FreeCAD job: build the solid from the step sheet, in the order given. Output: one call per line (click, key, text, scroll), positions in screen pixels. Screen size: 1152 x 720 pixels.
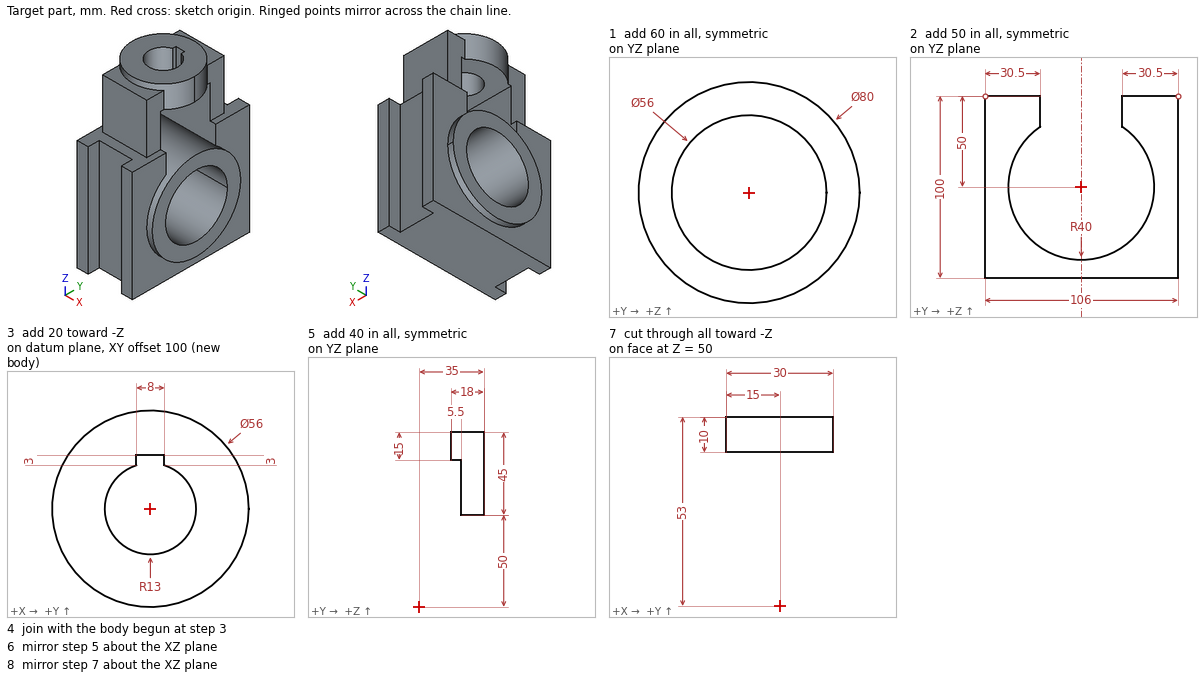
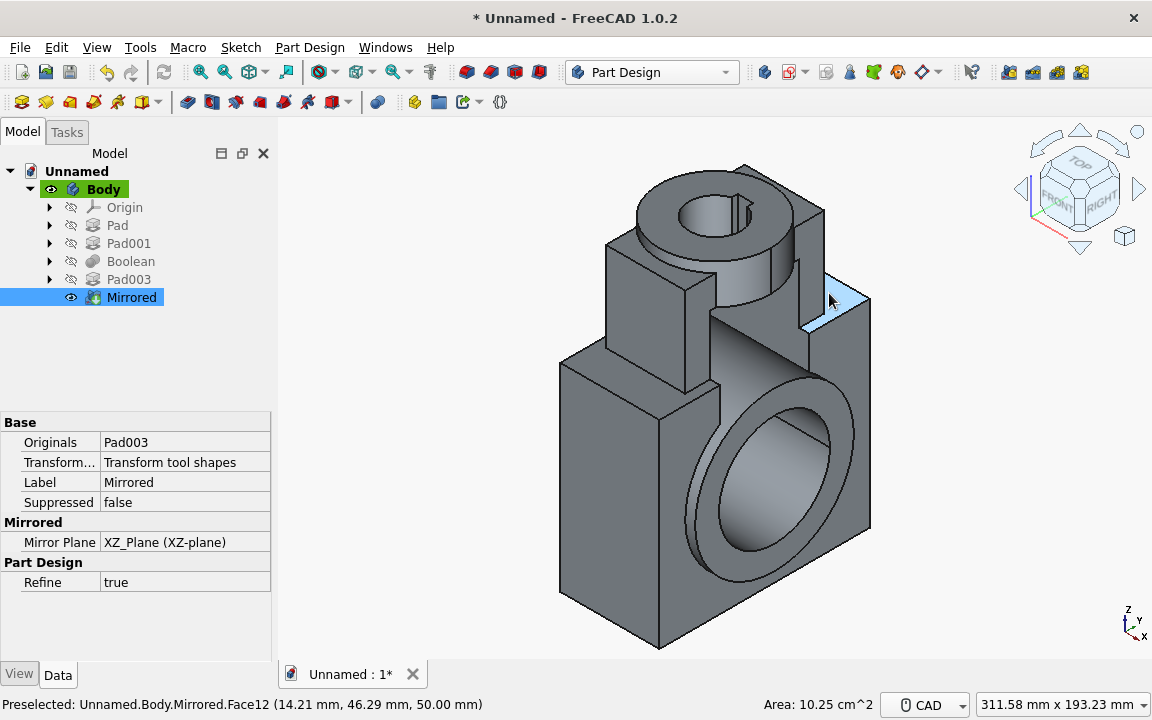
click(790, 72)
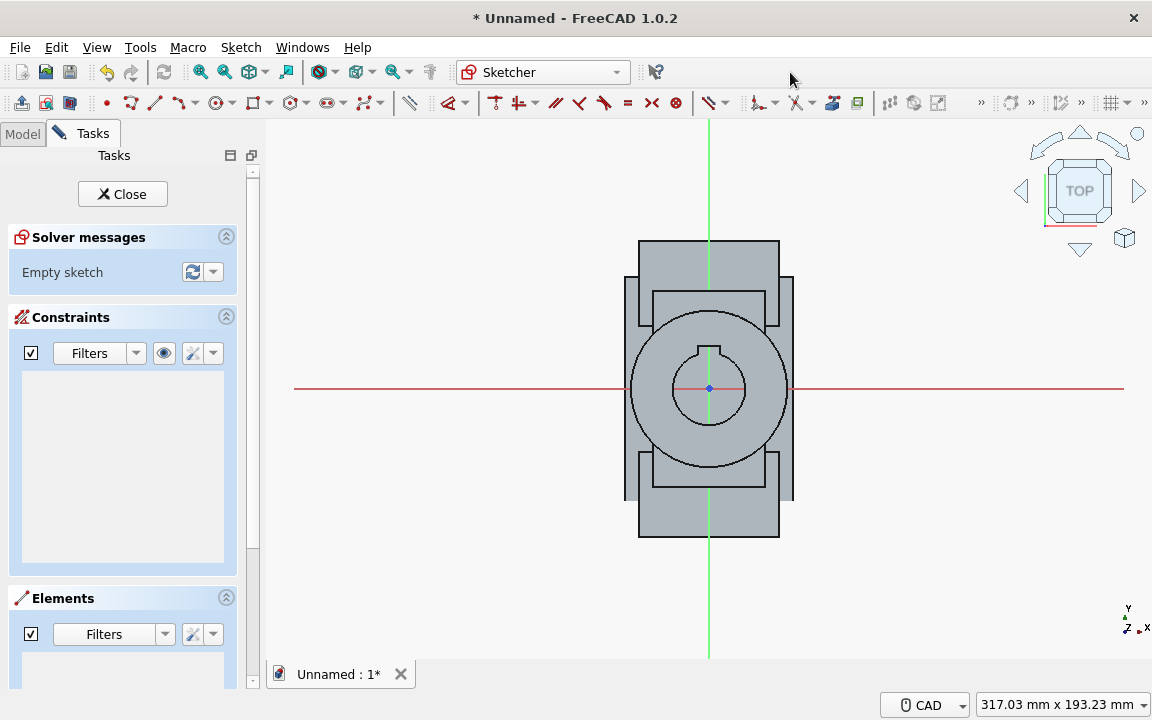
click(70, 104)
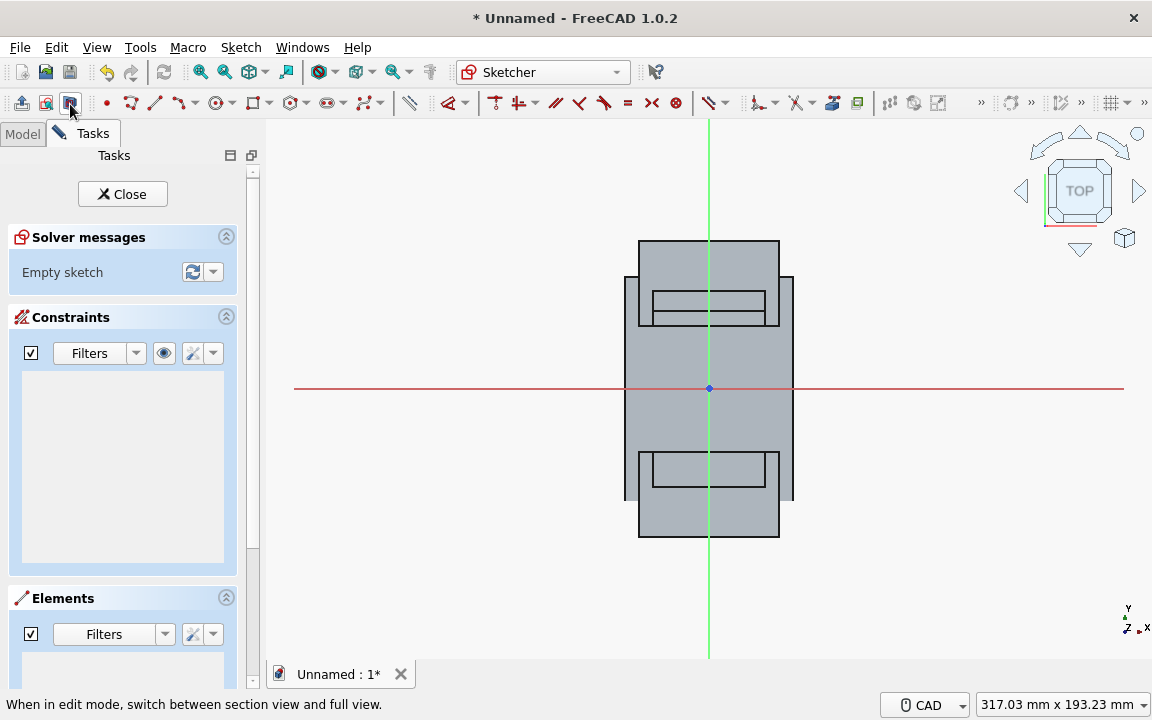
scroll(765, 255, up, 4)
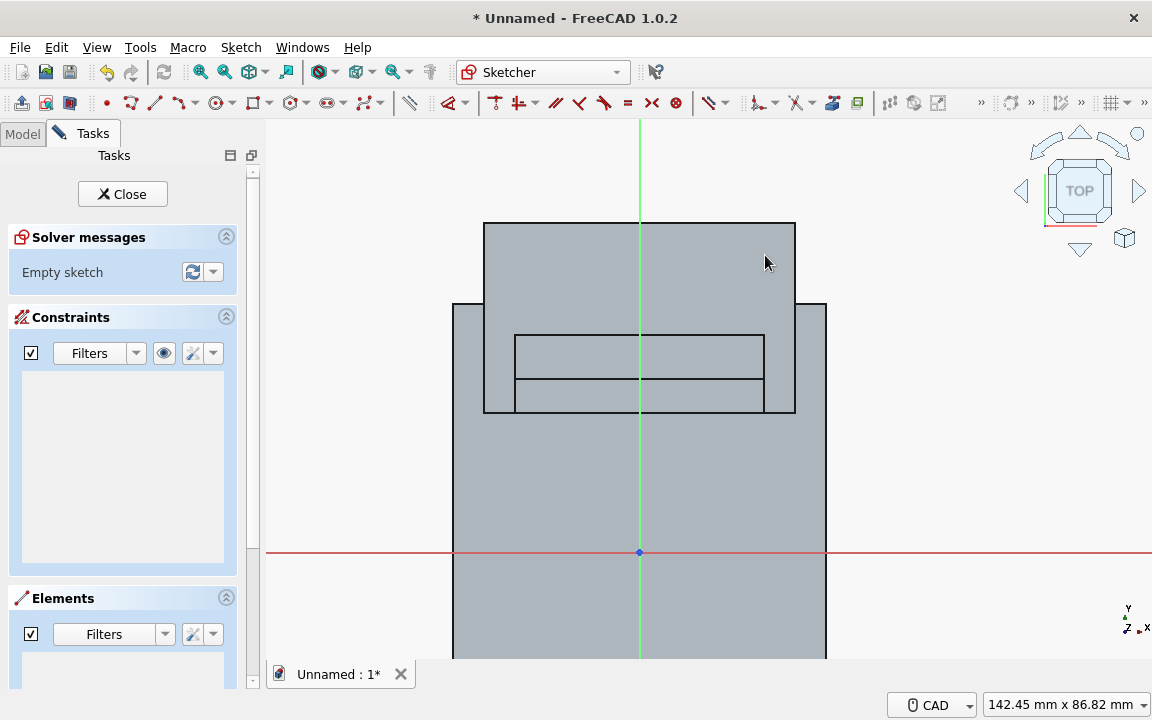
click(254, 104)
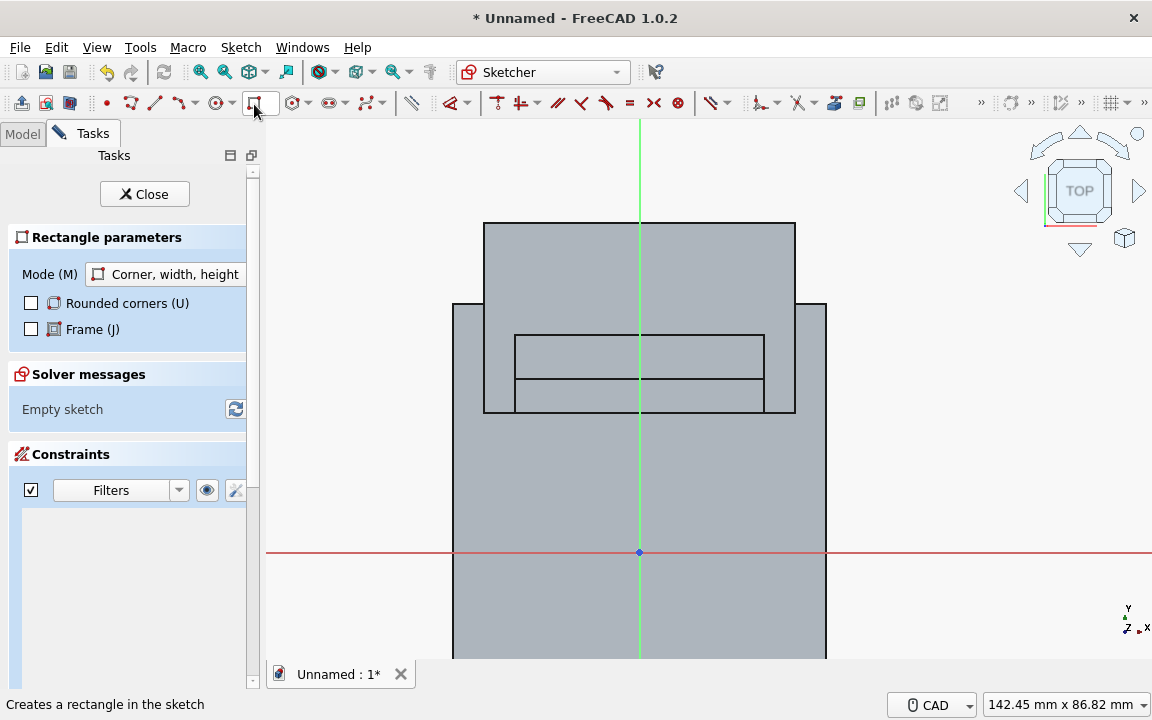
click(546, 223)
click(733, 285)
key(Escape)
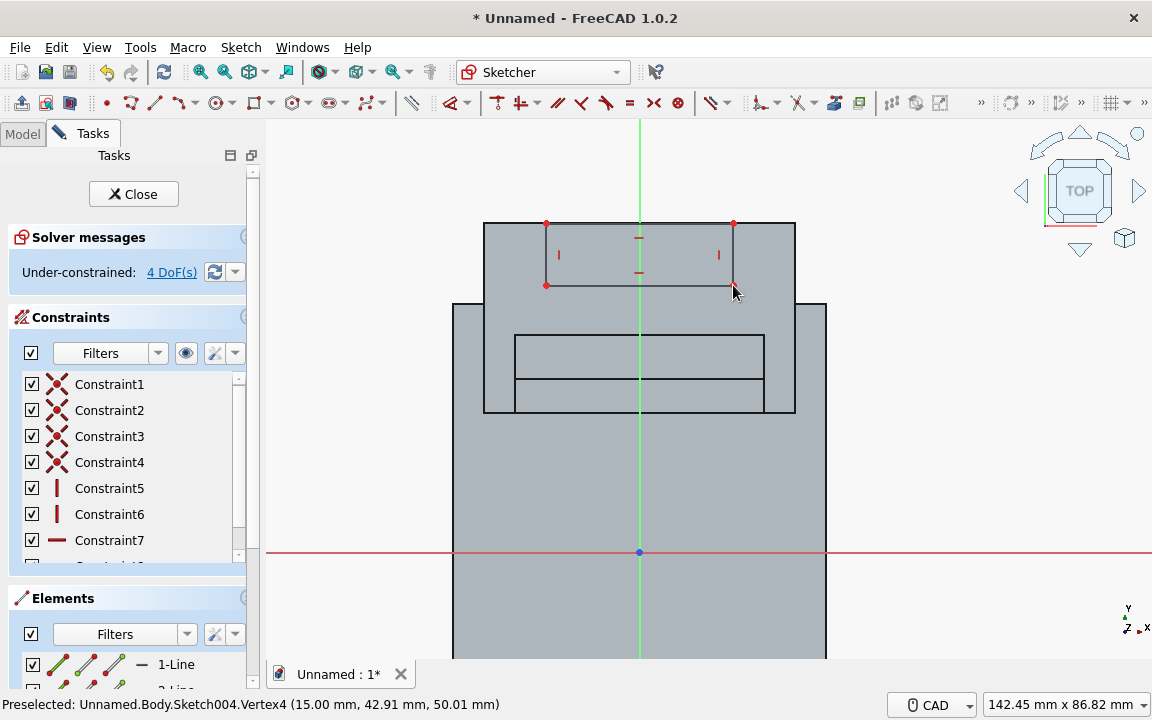
click(450, 104)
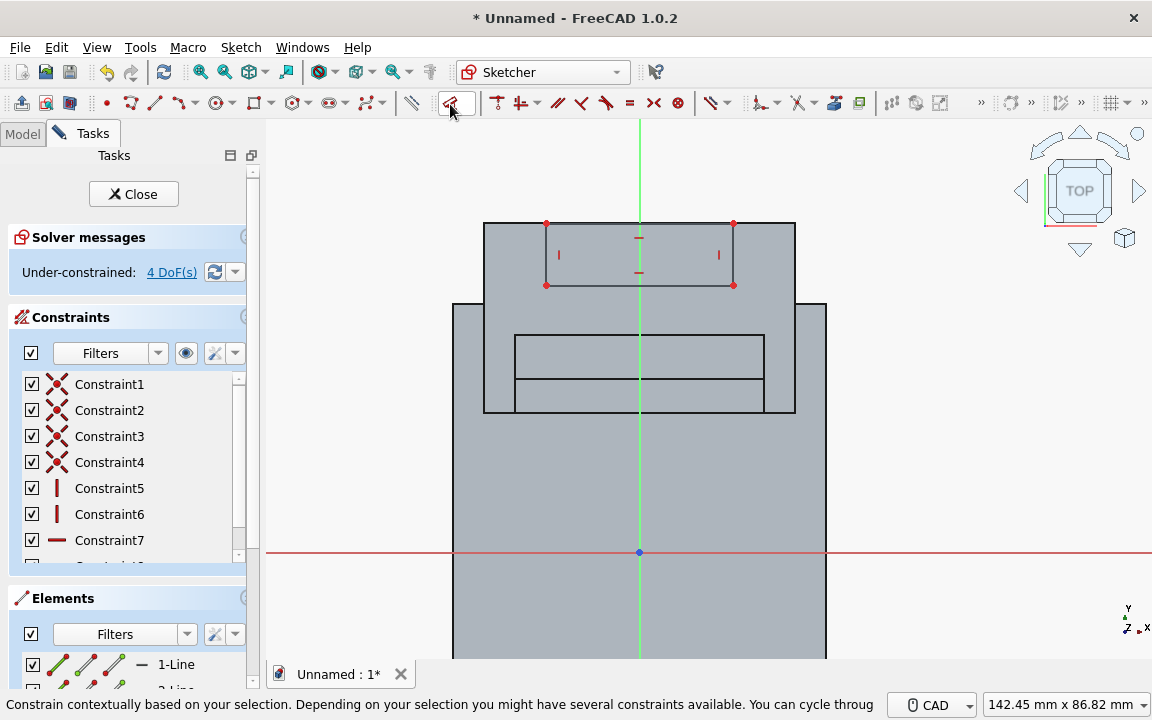
click(546, 243)
click(512, 255)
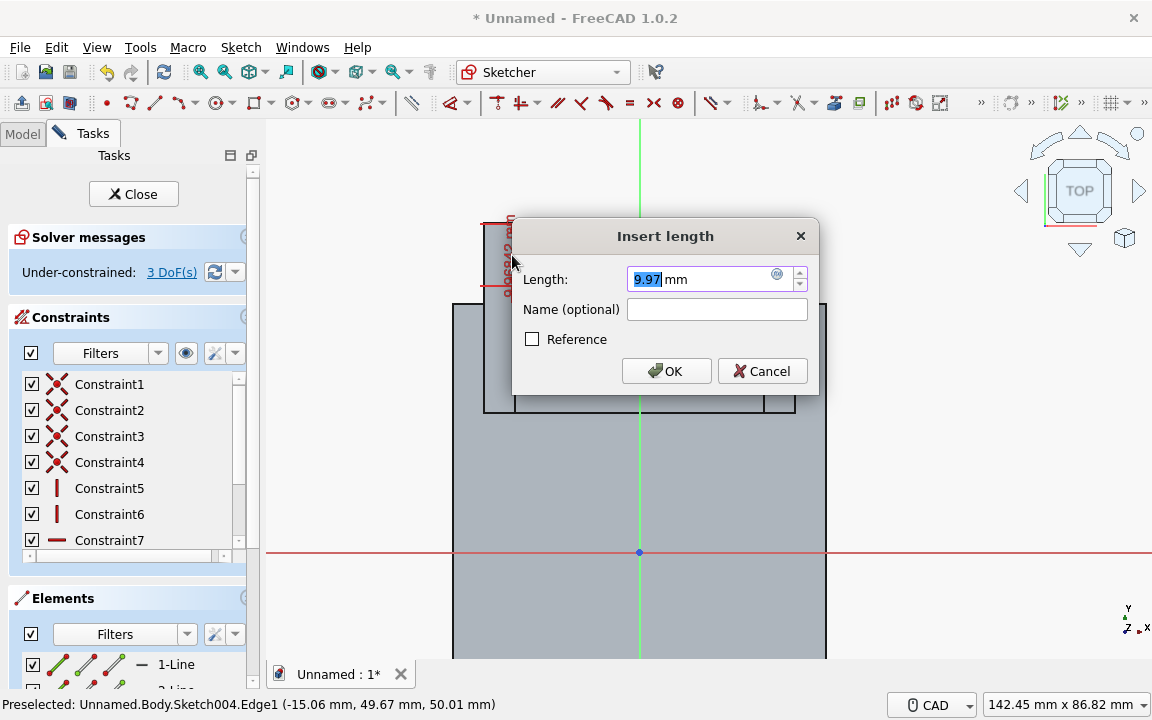
text(10)
key(Return)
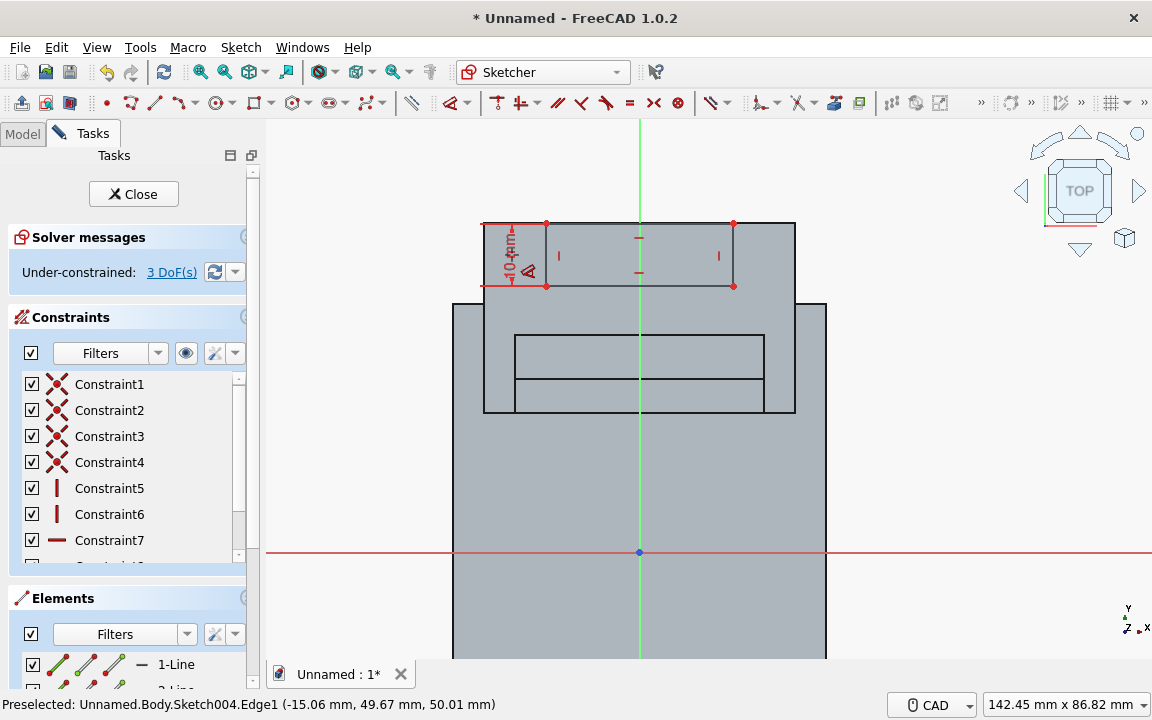
click(602, 286)
click(596, 252)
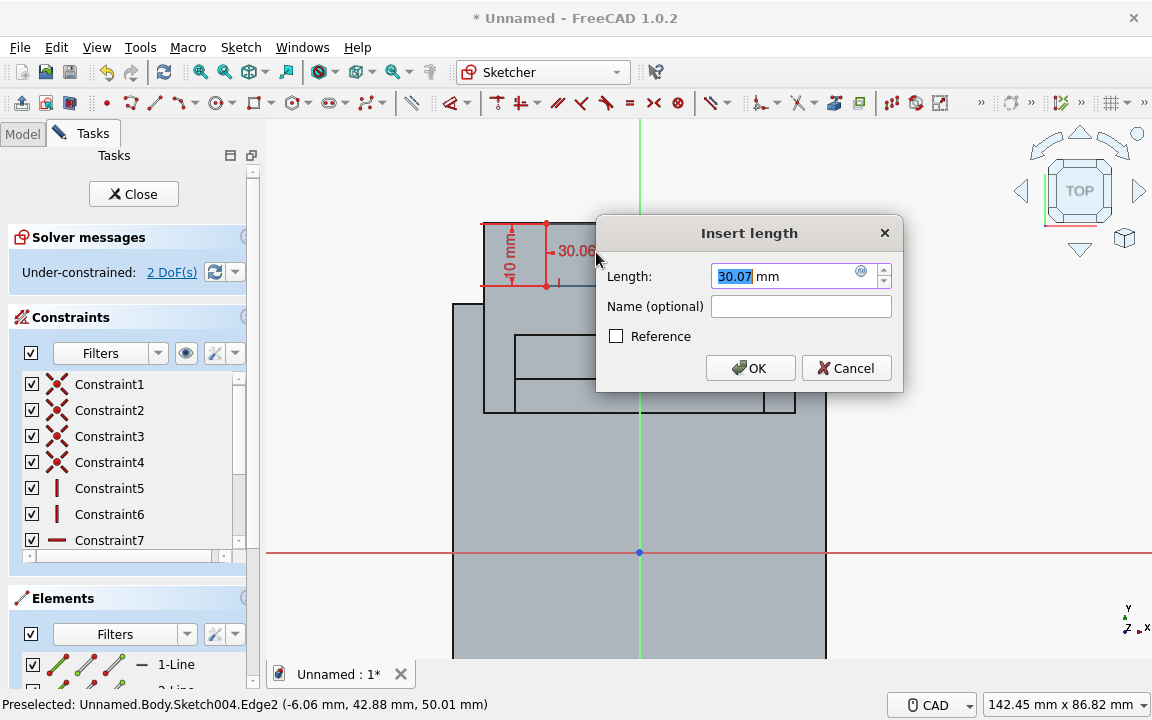
text(30)
key(Return)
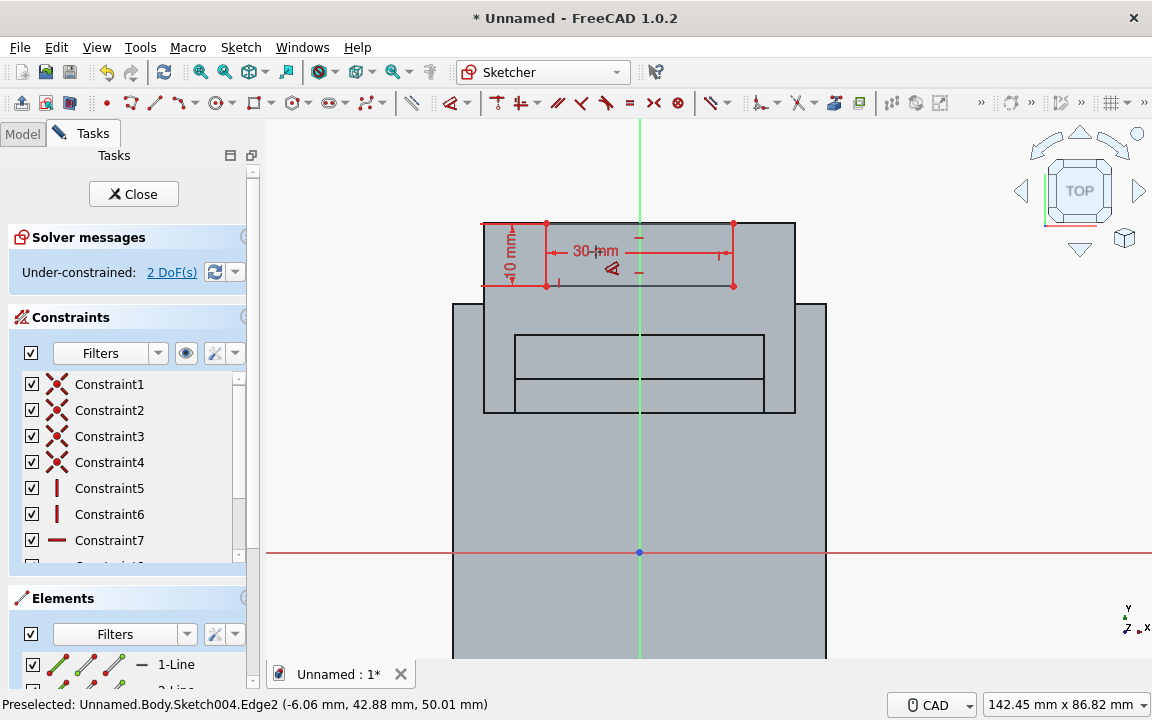
click(546, 224)
click(593, 587)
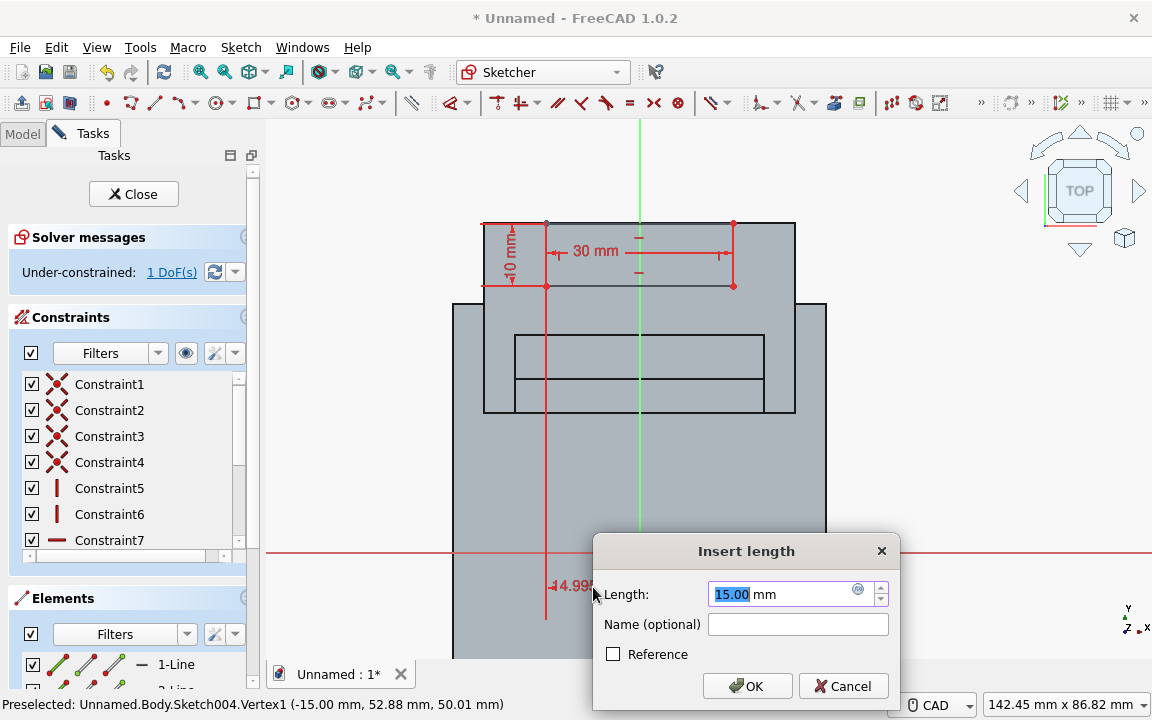
text(15)
key(Return)